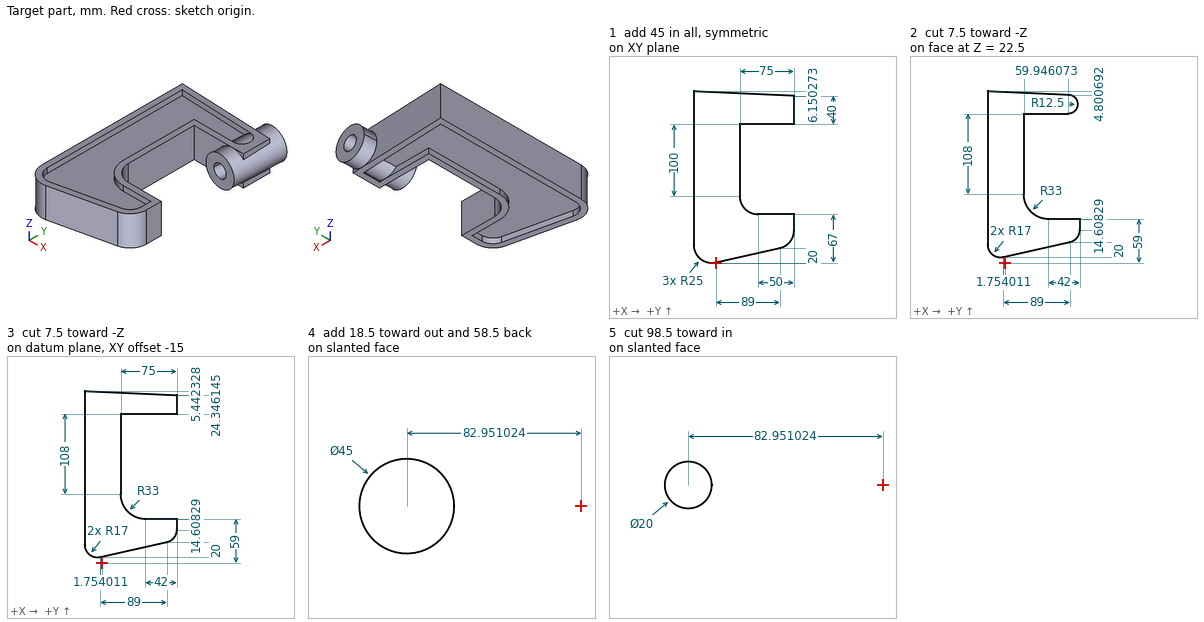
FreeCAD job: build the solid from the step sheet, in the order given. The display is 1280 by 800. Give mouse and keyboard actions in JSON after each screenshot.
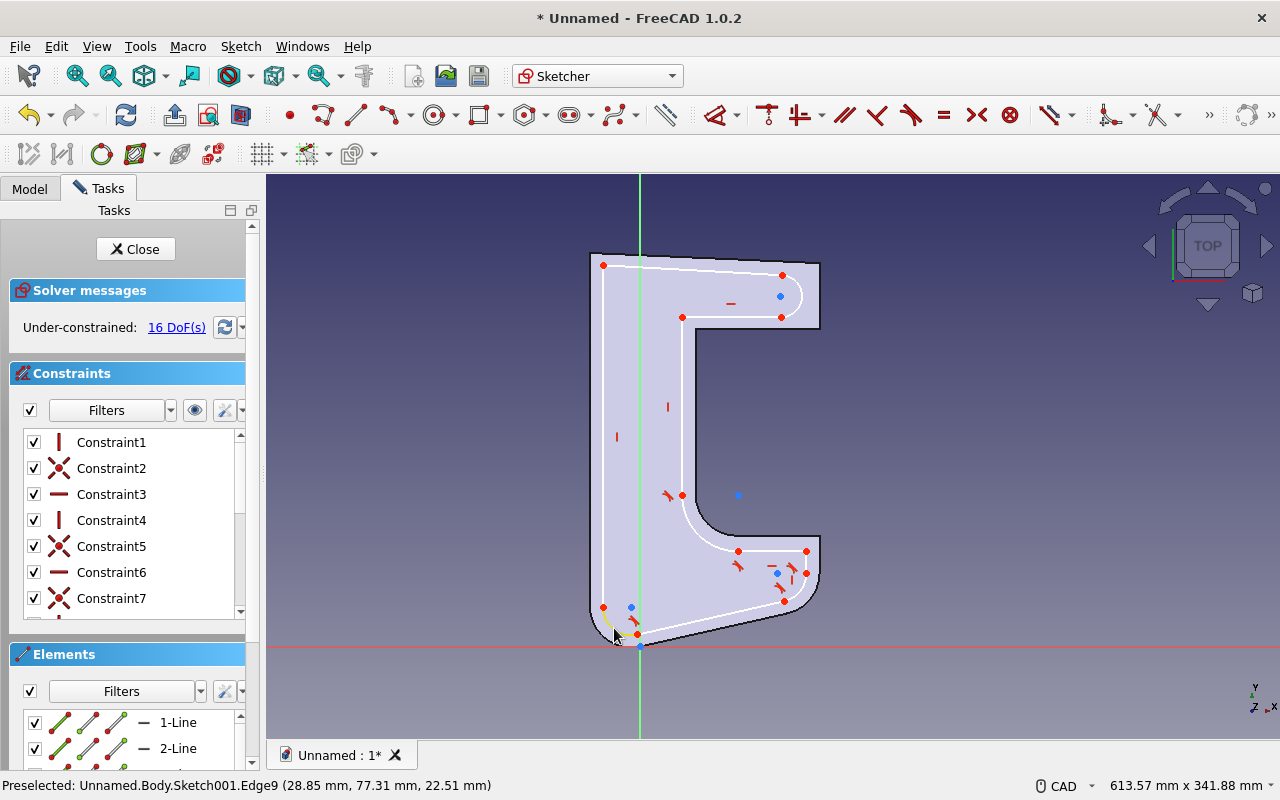
{"action": "left_click", "coordinate": [712, 317]}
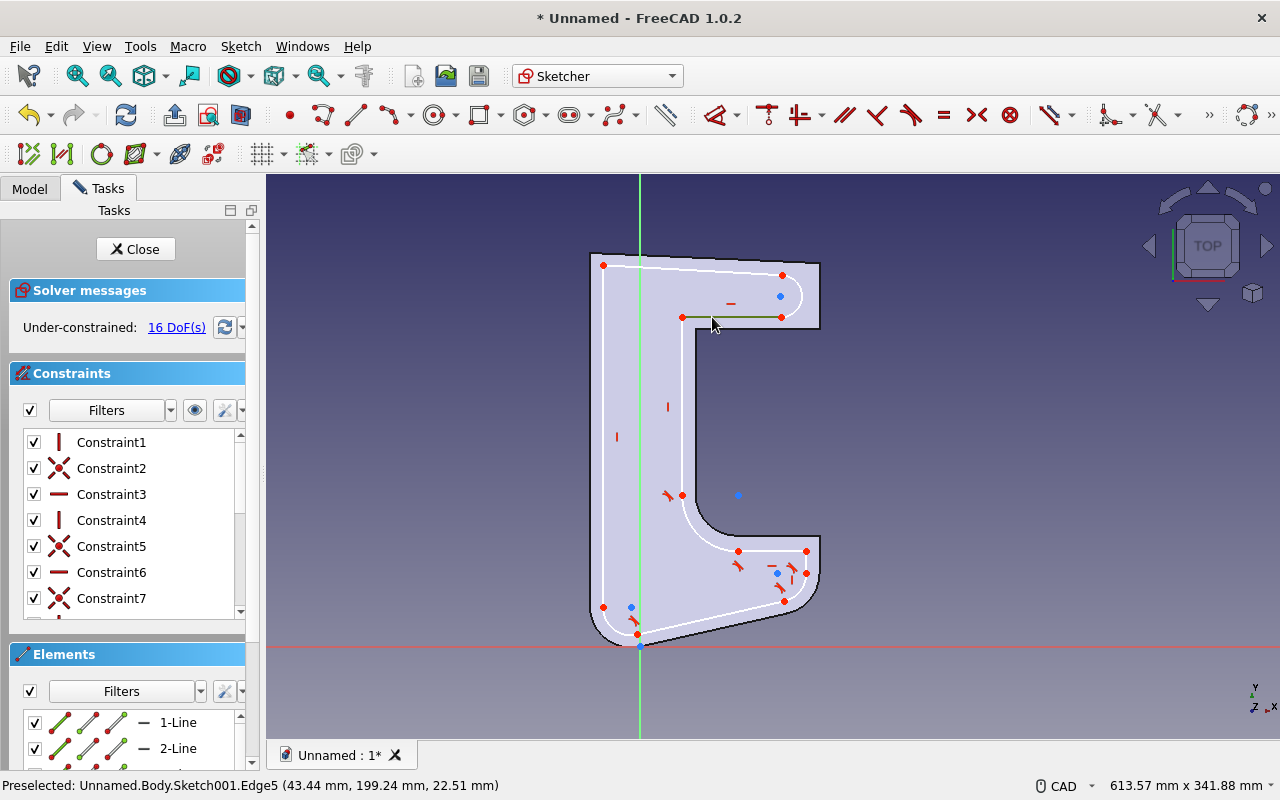
{"action": "left_click", "coordinate": [798, 309]}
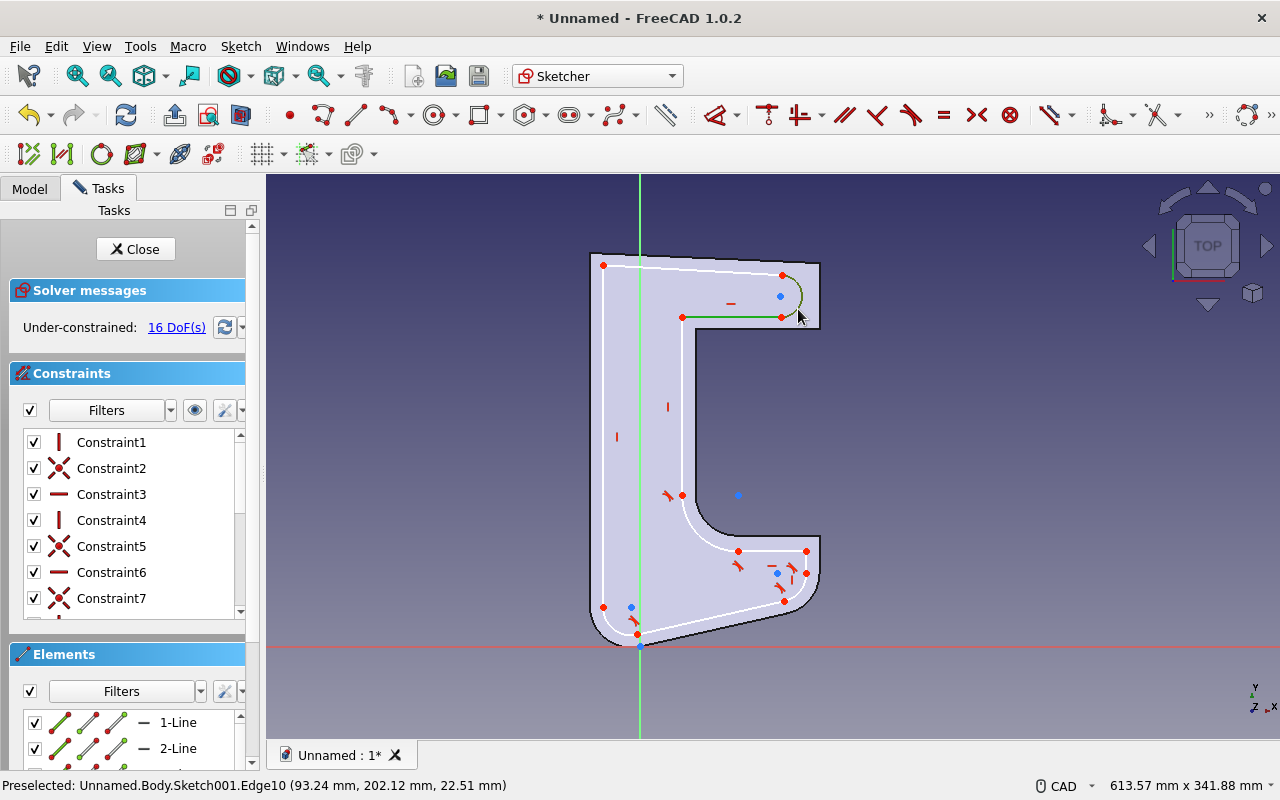
{"action": "left_click", "coordinate": [911, 116]}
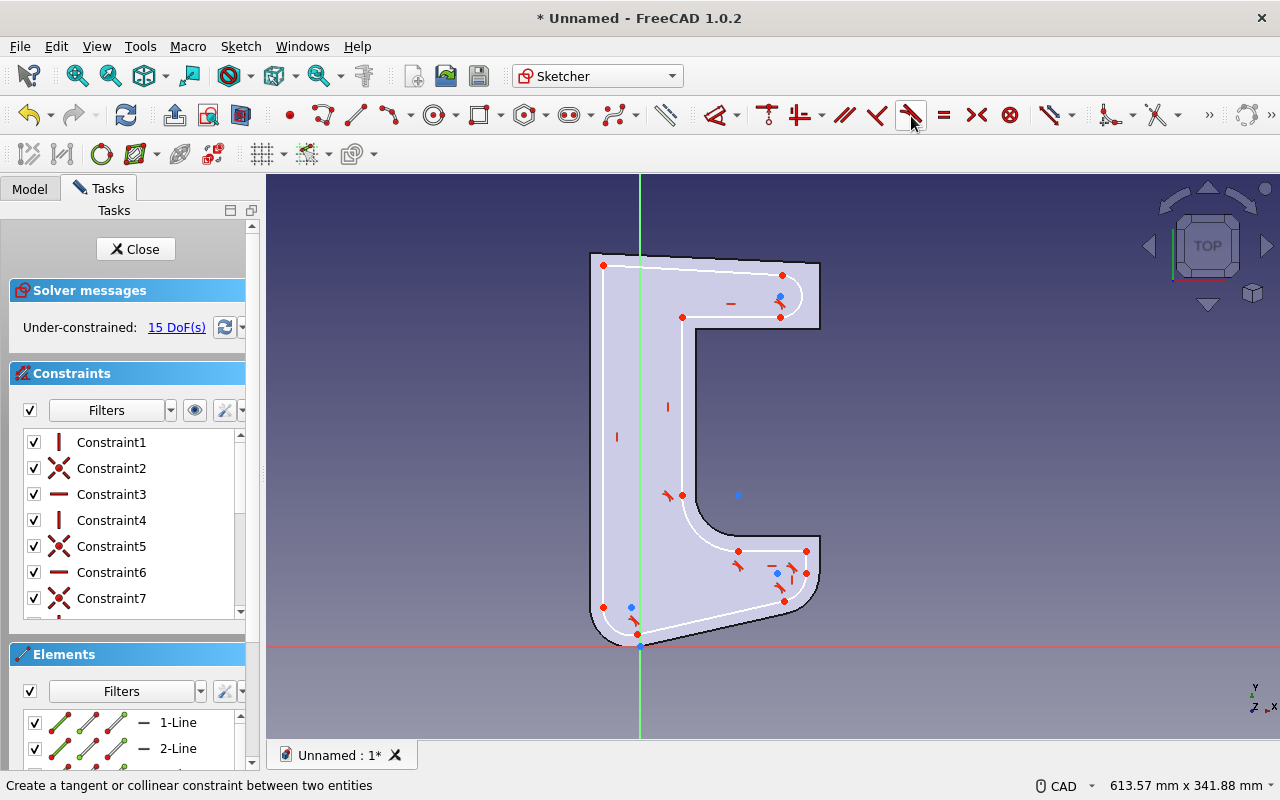
{"action": "left_click", "coordinate": [728, 272]}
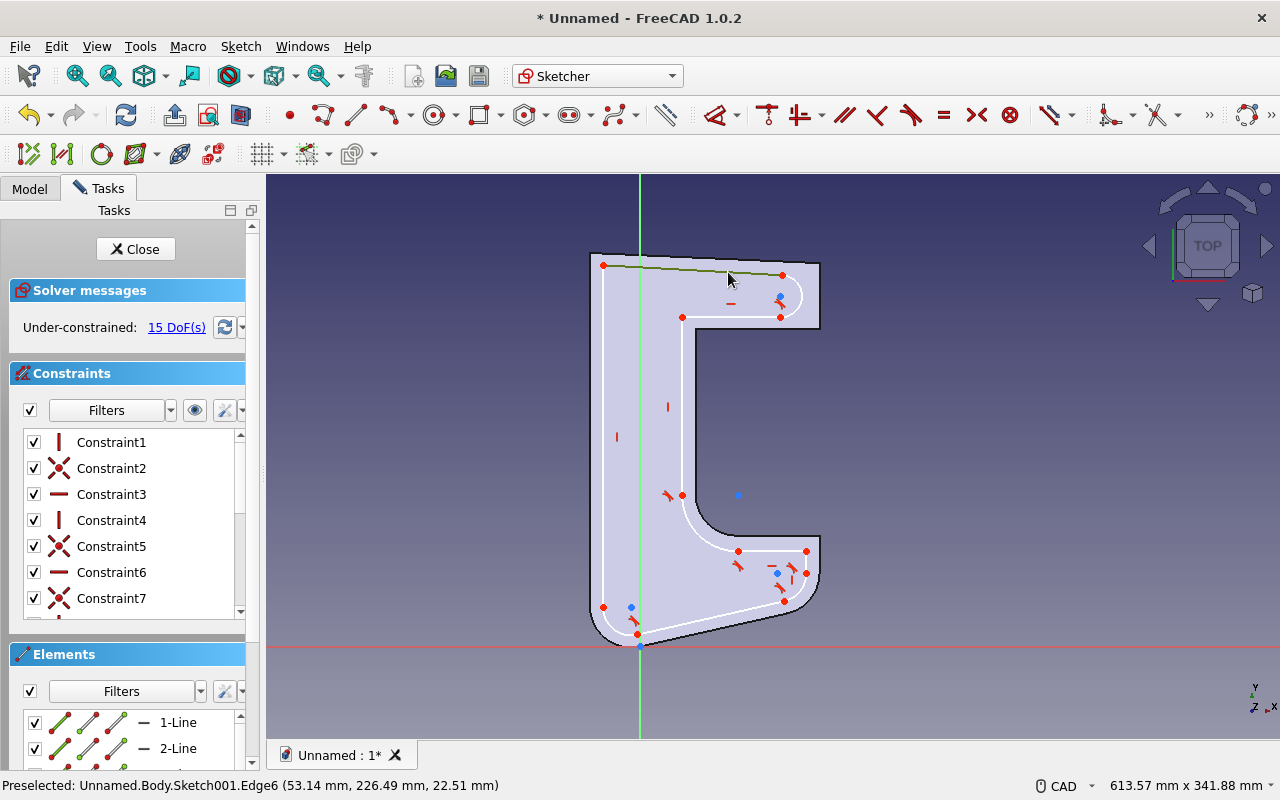
{"action": "left_click", "coordinate": [798, 309]}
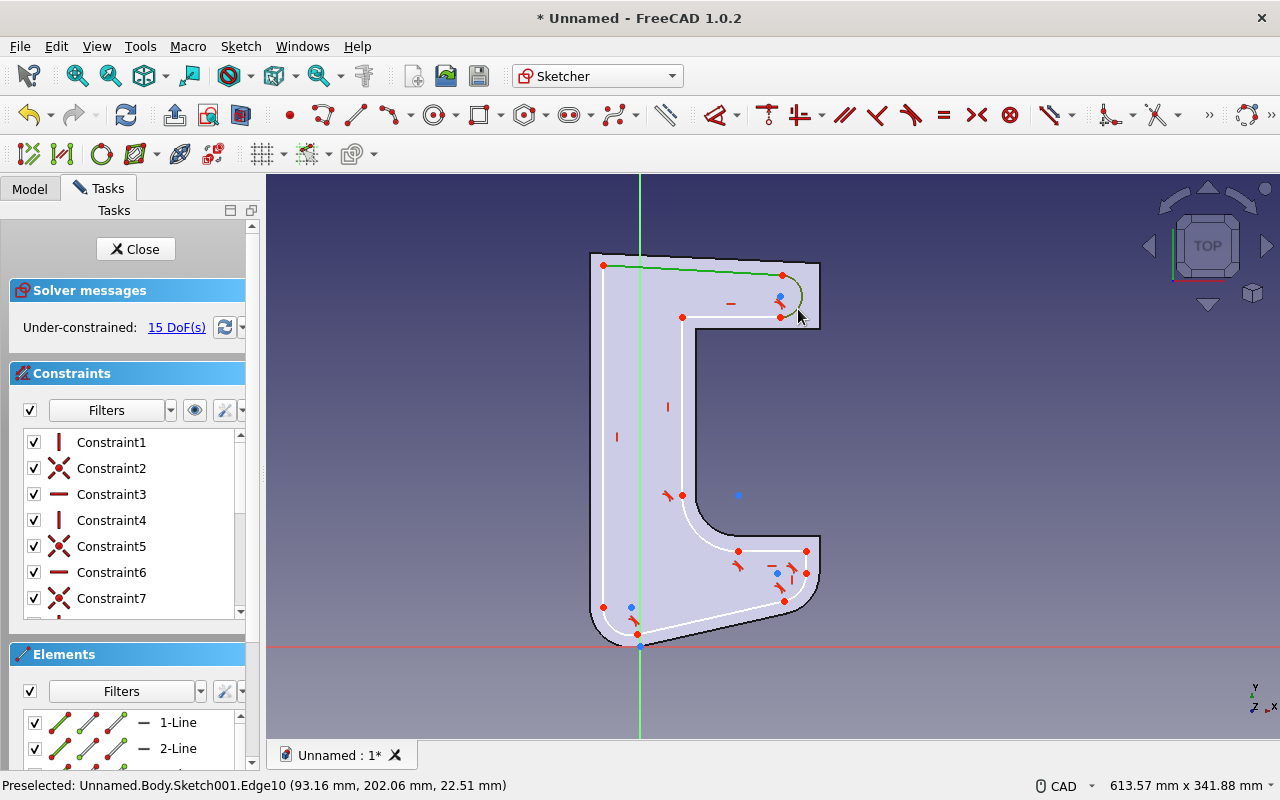
{"action": "left_click", "coordinate": [911, 116]}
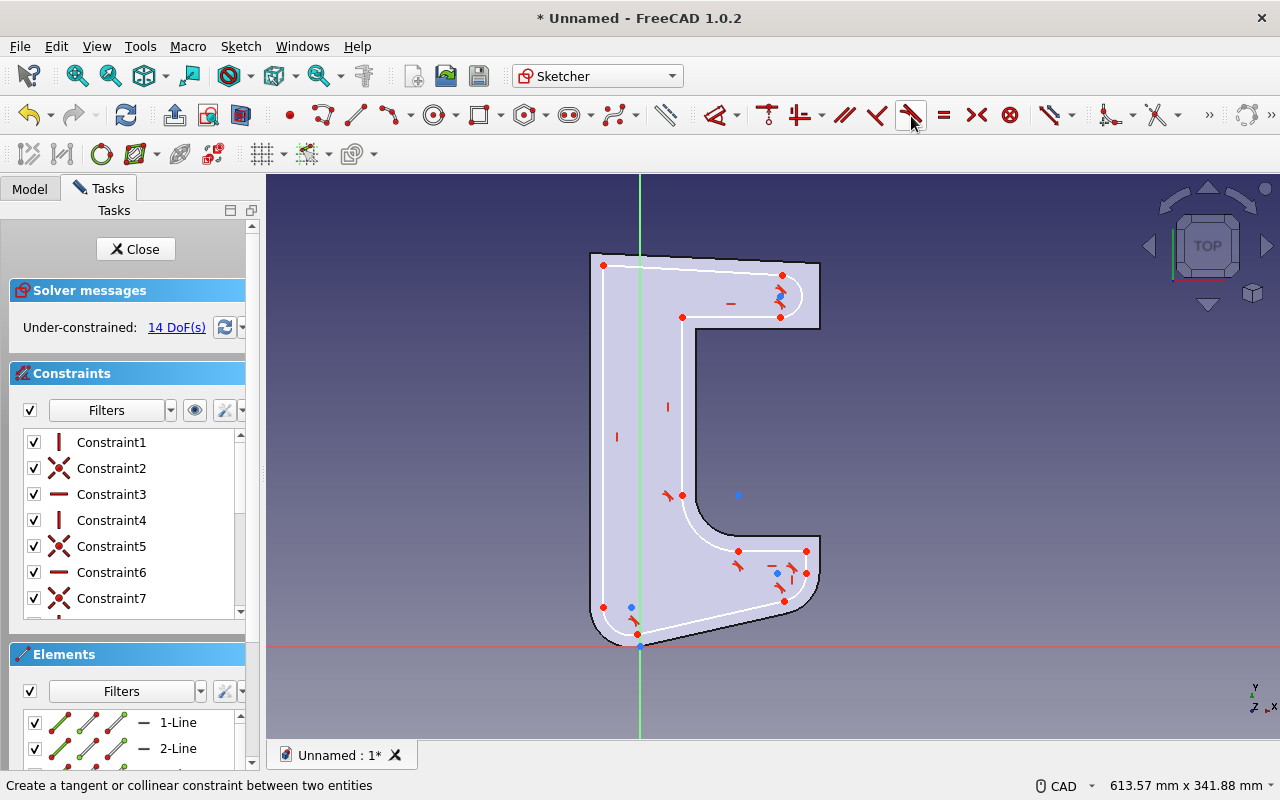
{"action": "left_click", "coordinate": [603, 368]}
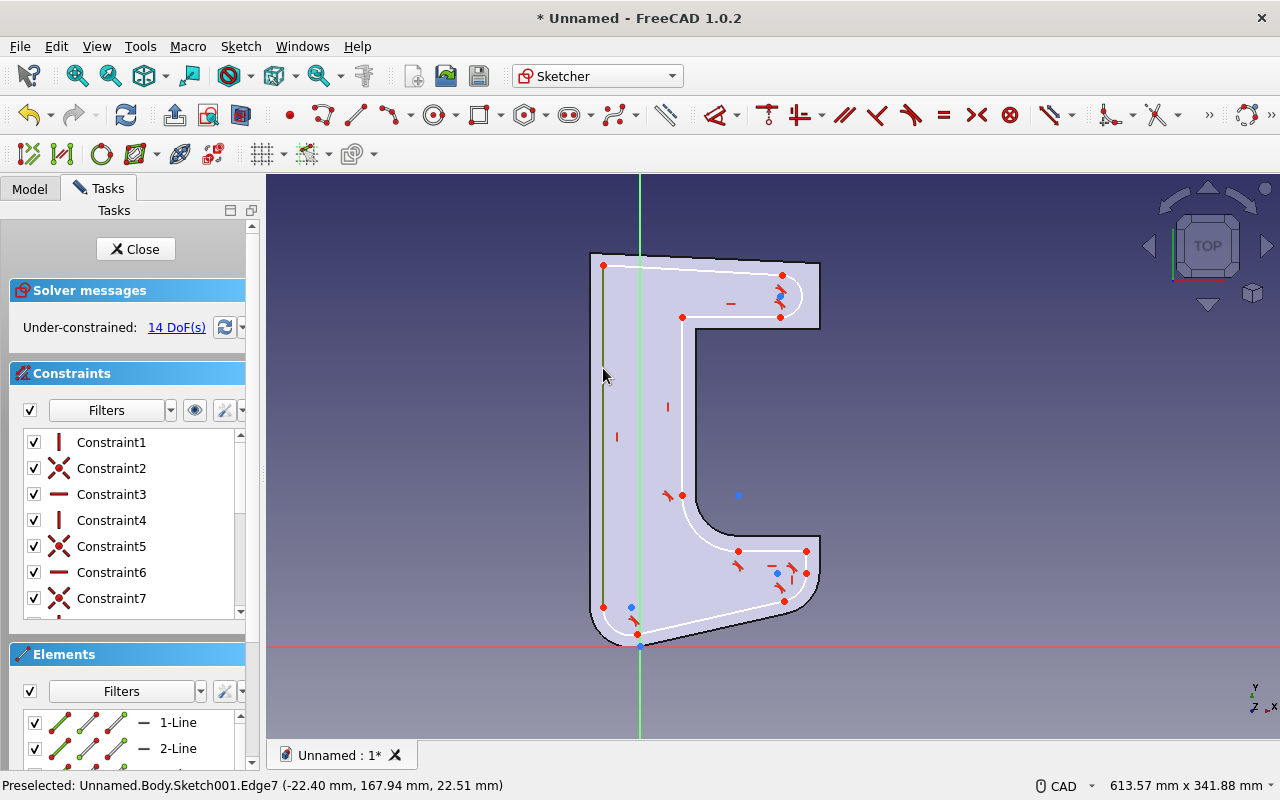
{"action": "left_click", "coordinate": [607, 622]}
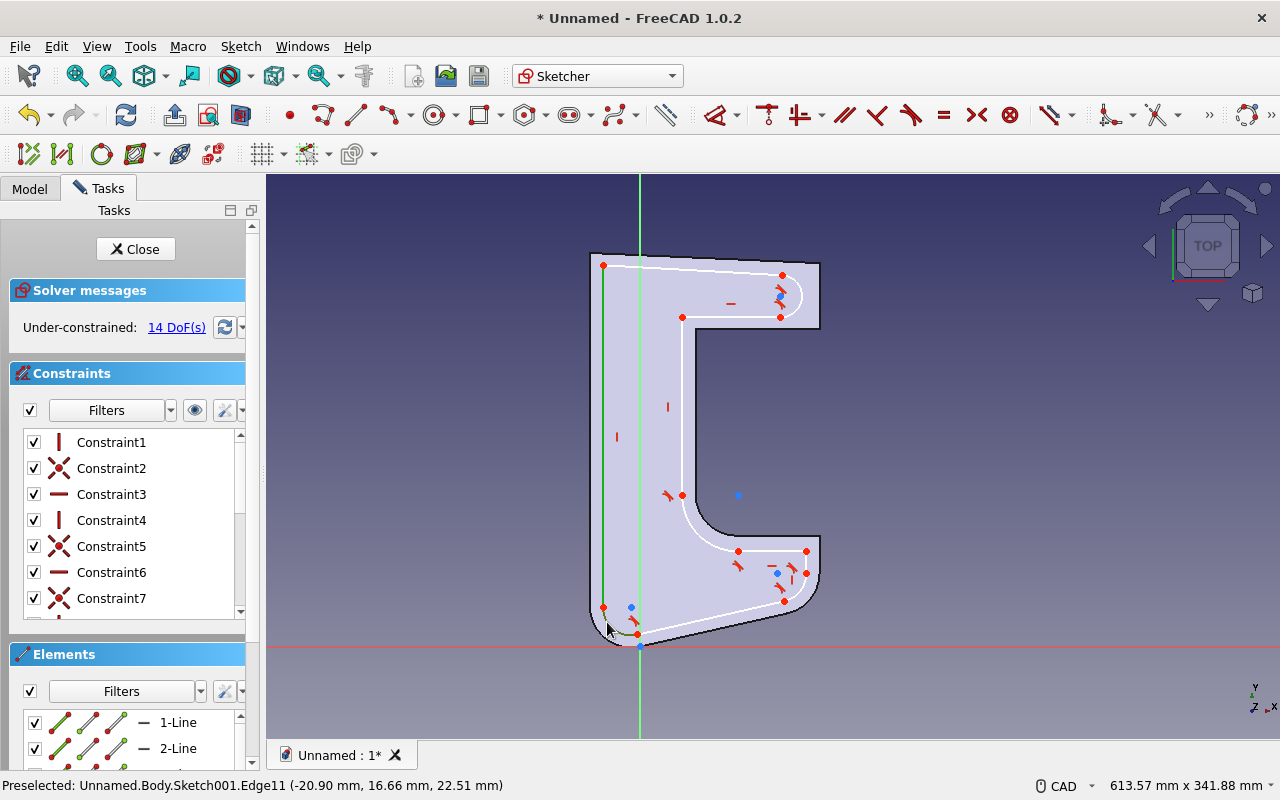
{"action": "left_click", "coordinate": [911, 116]}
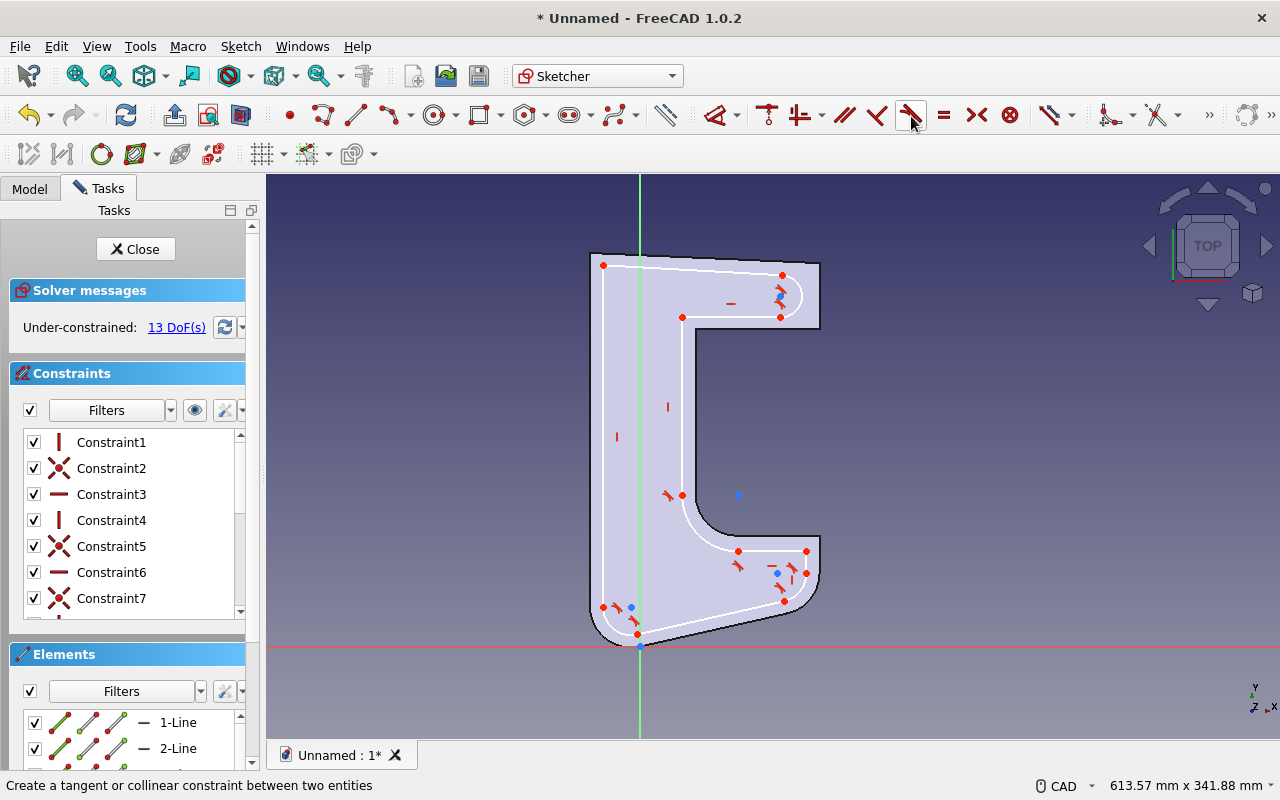
{"action": "left_click", "coordinate": [794, 597]}